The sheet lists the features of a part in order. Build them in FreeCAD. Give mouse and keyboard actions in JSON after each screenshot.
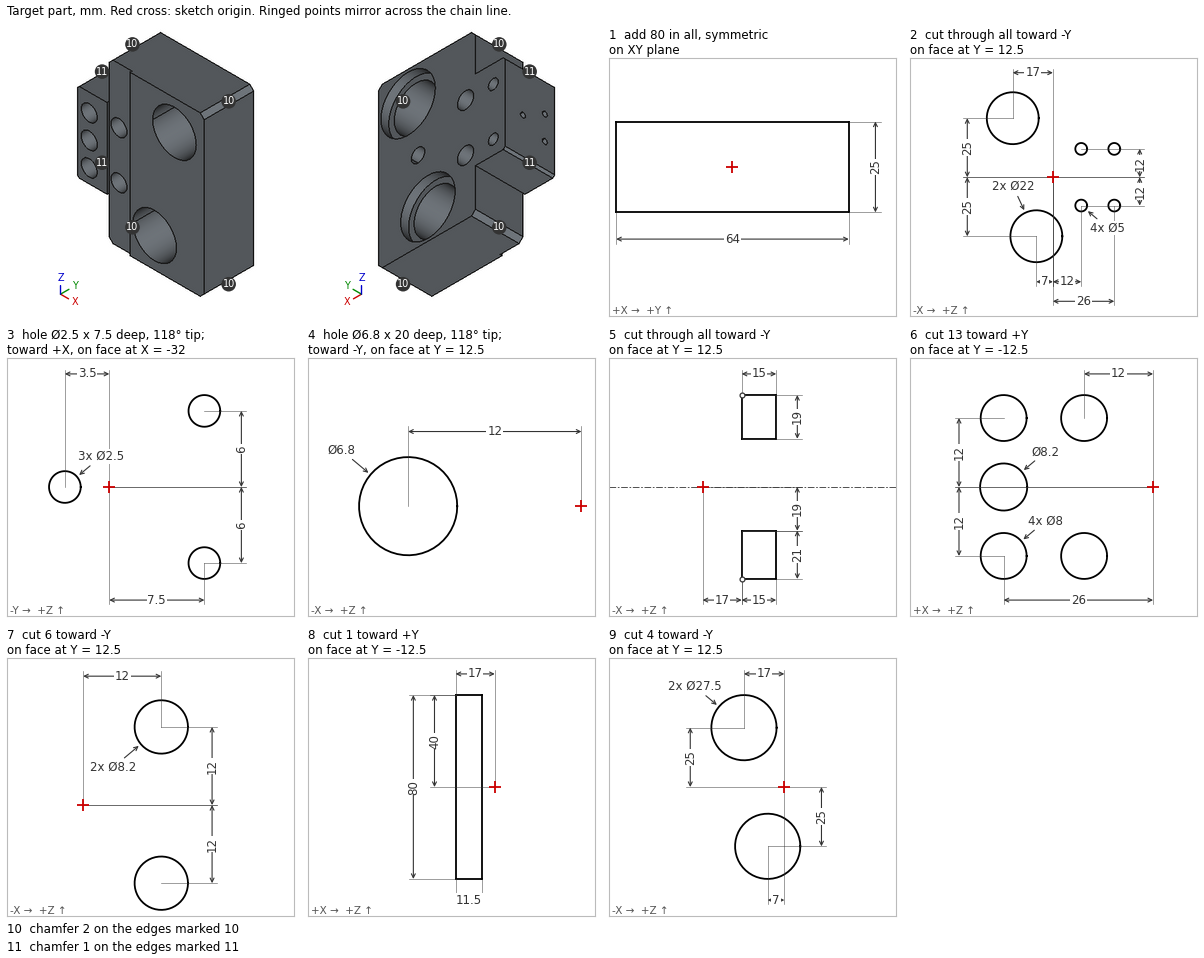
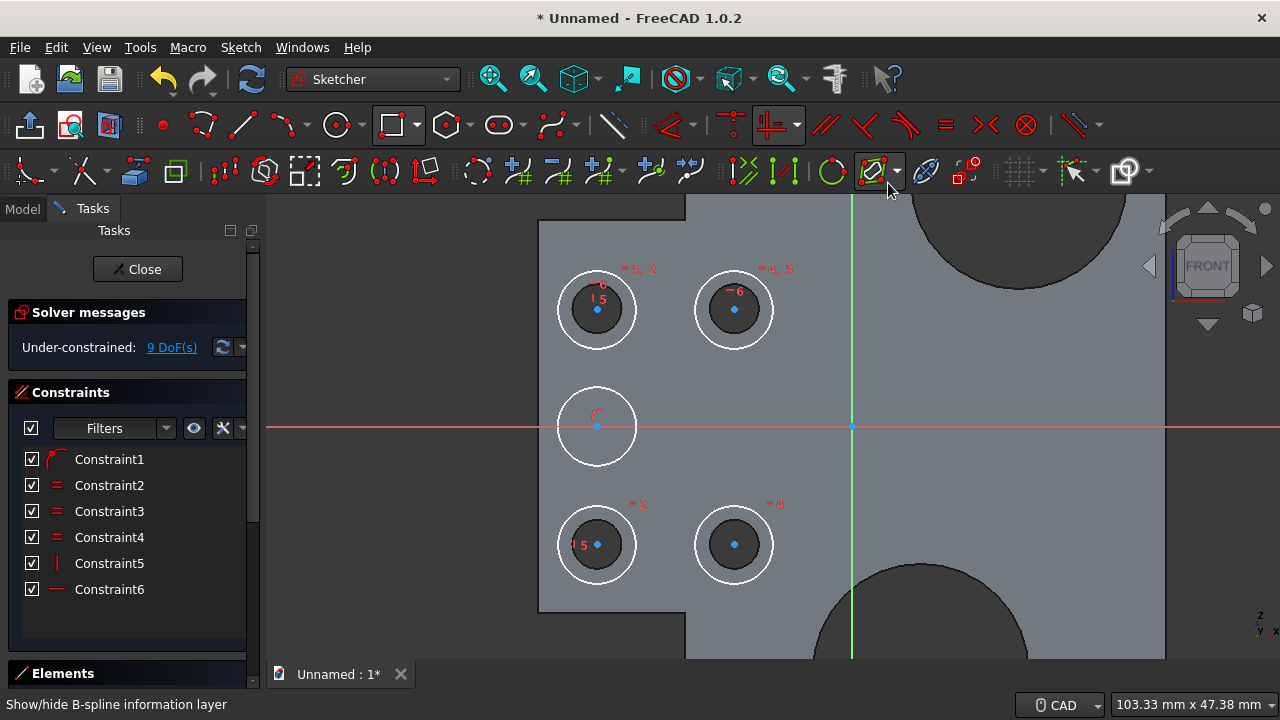
{"action": "left_click", "coordinate": [734, 310]}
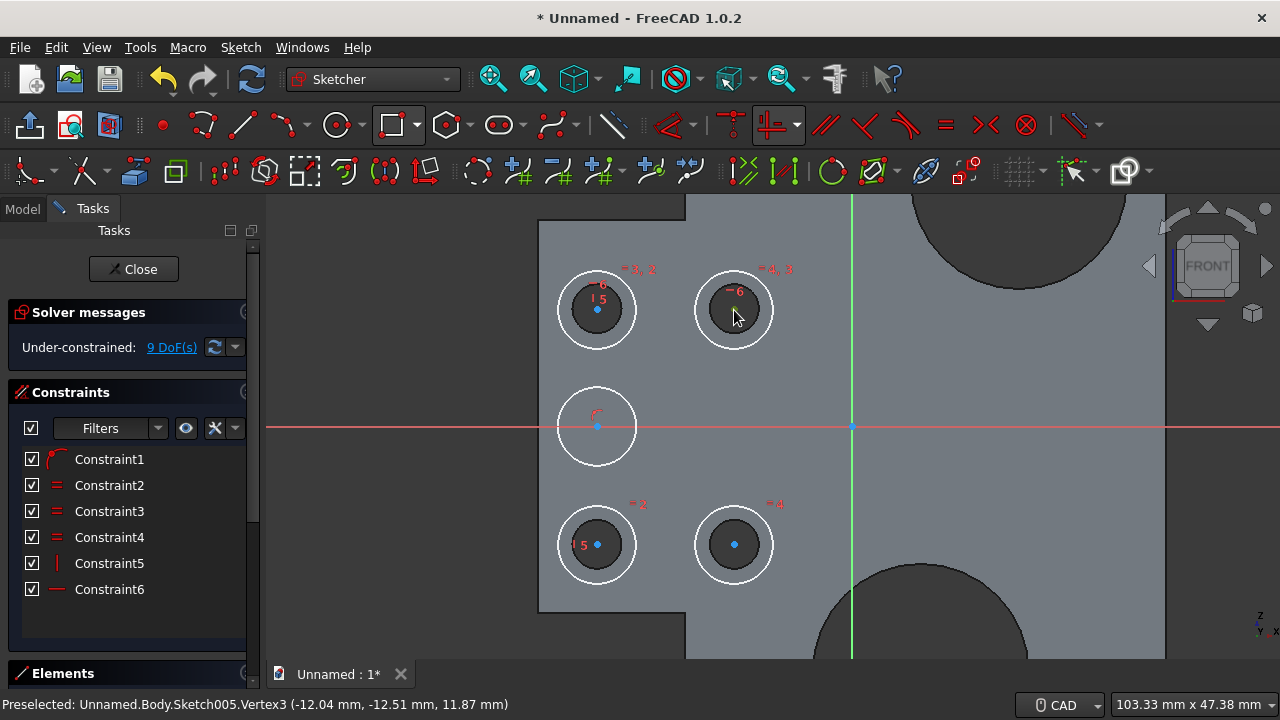
{"action": "left_click", "coordinate": [734, 545]}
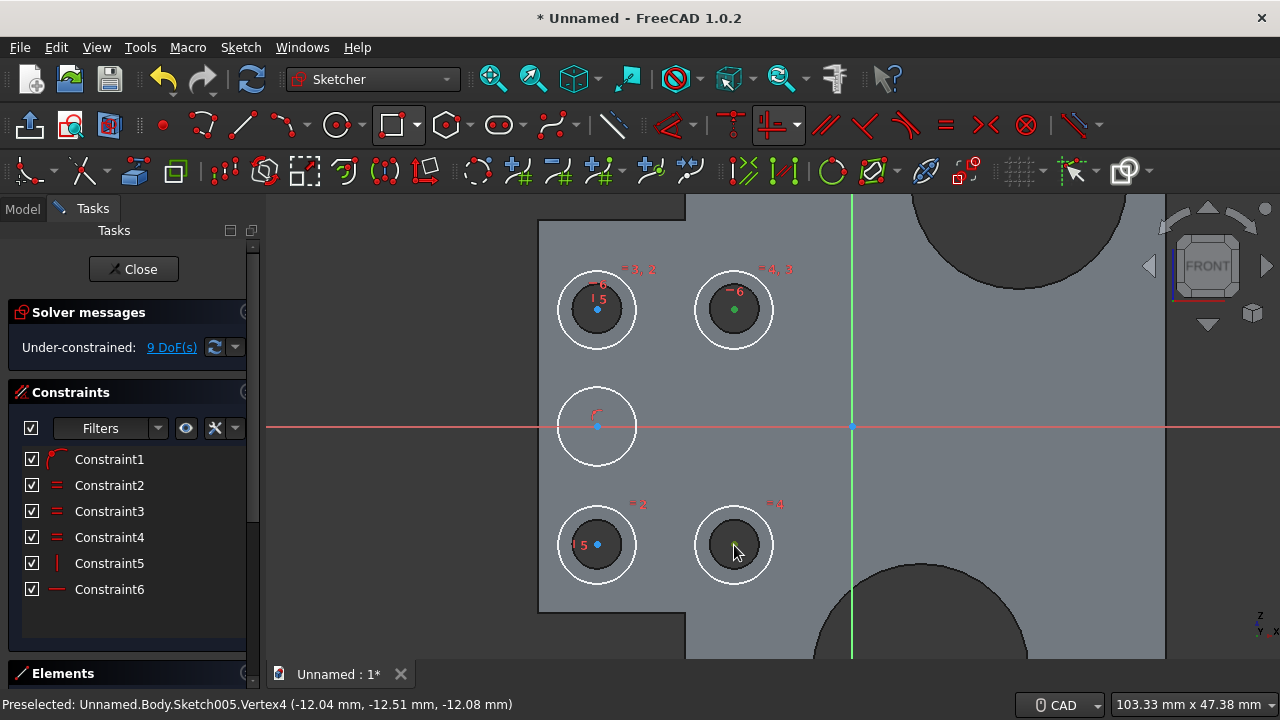
{"action": "left_click", "coordinate": [800, 126]}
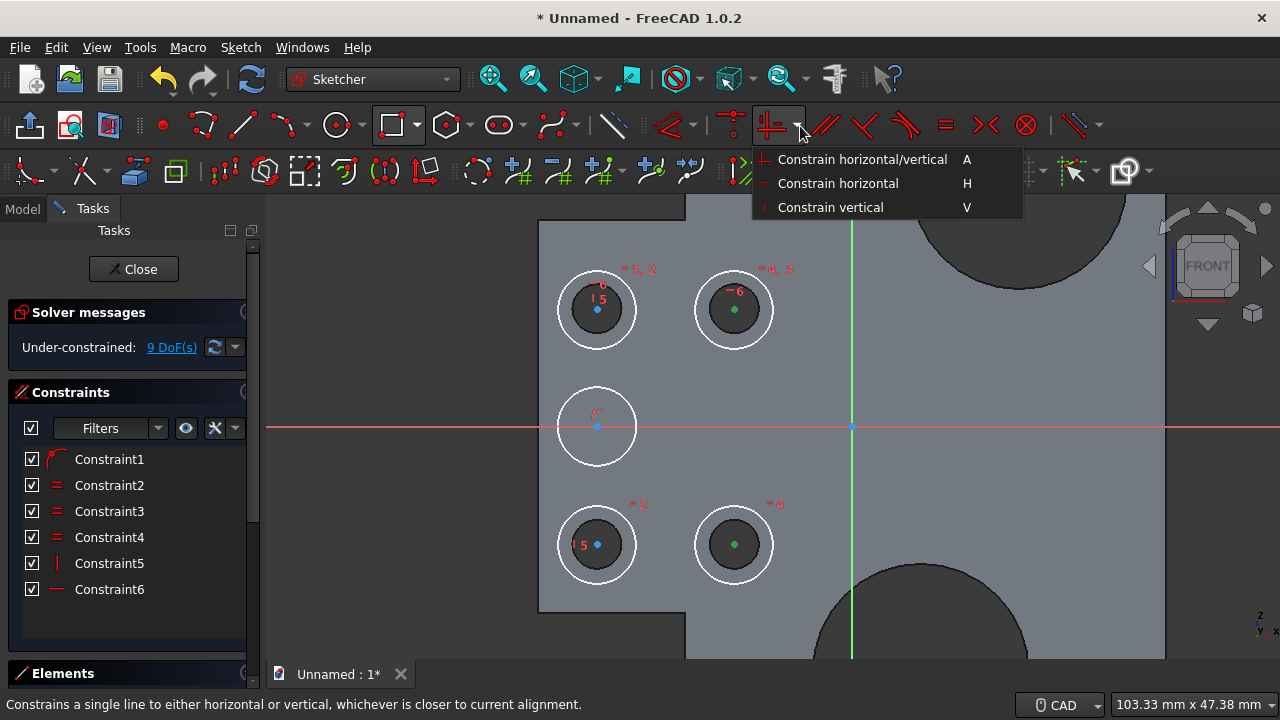
{"action": "left_click", "coordinate": [888, 207]}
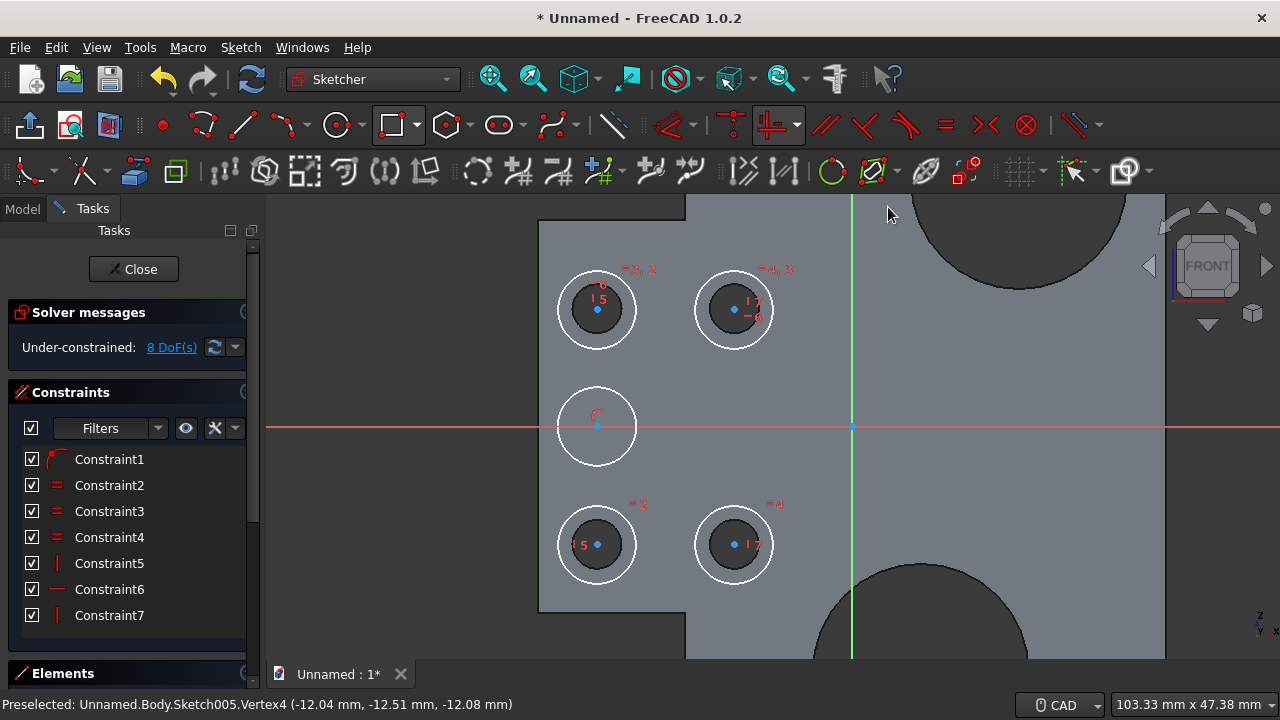
{"action": "left_click", "coordinate": [597, 545]}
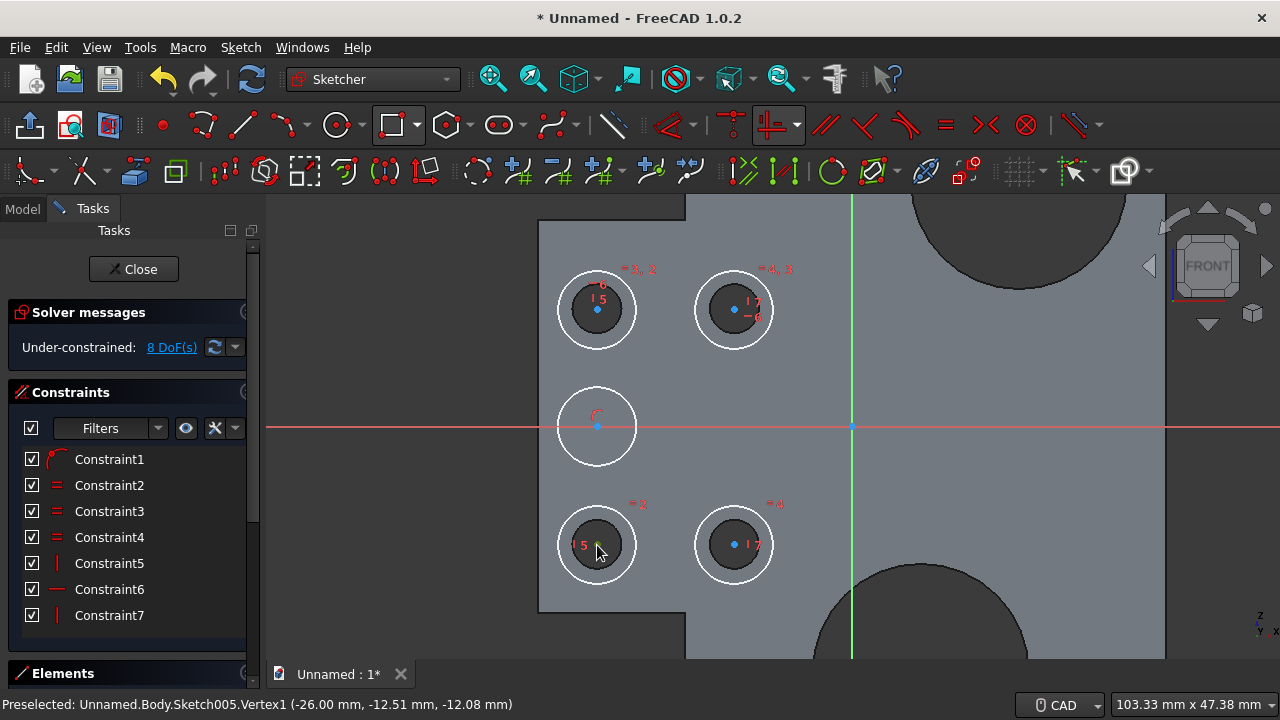
{"action": "left_click", "coordinate": [734, 545]}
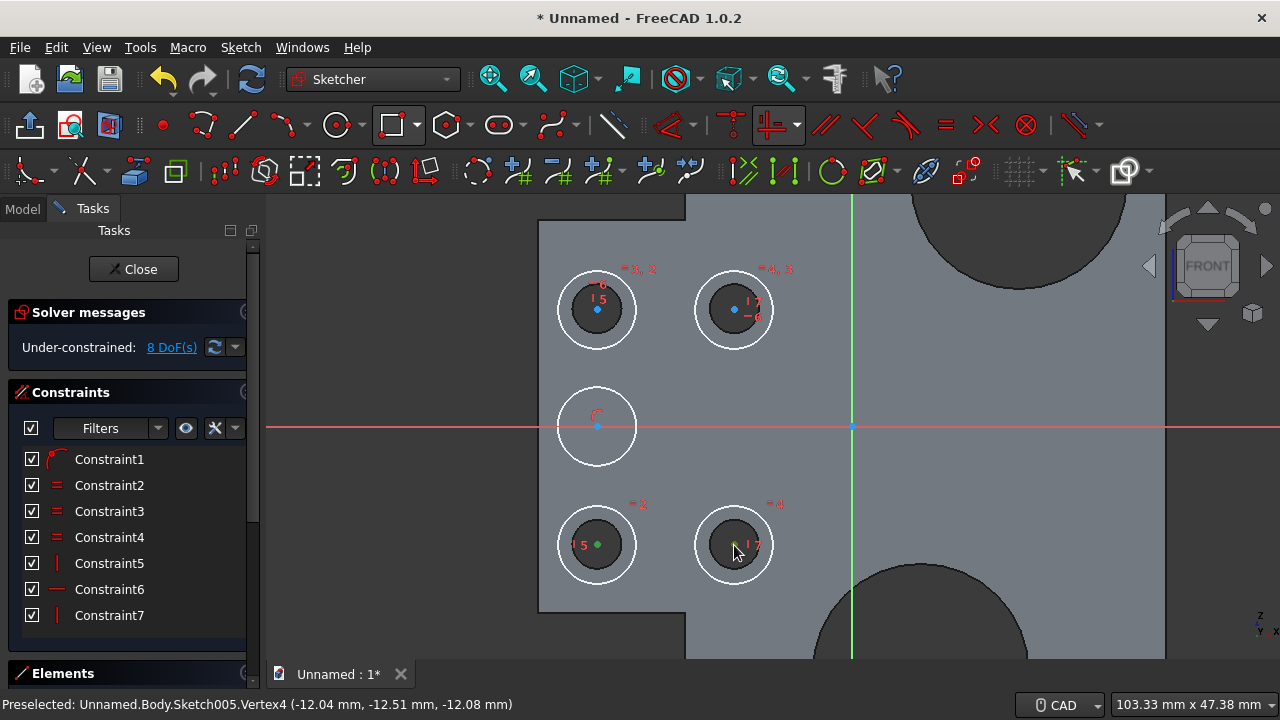
{"action": "left_click", "coordinate": [800, 126]}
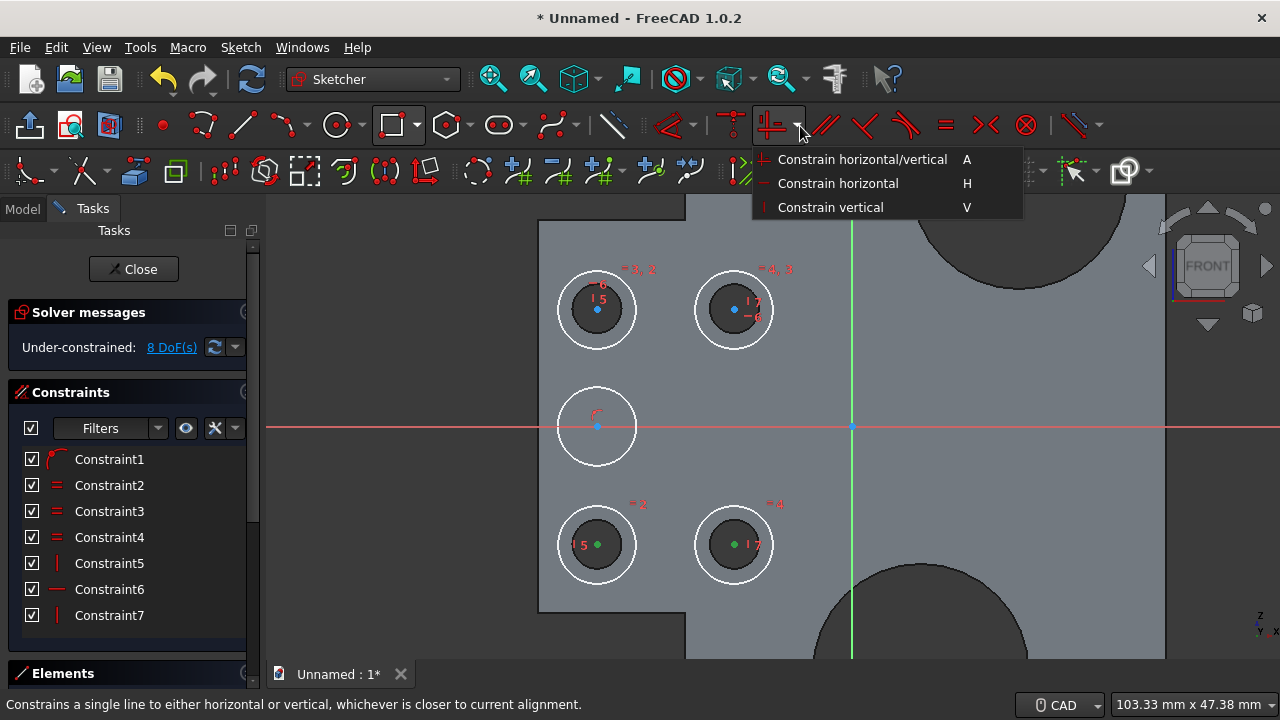
{"action": "left_click", "coordinate": [888, 183]}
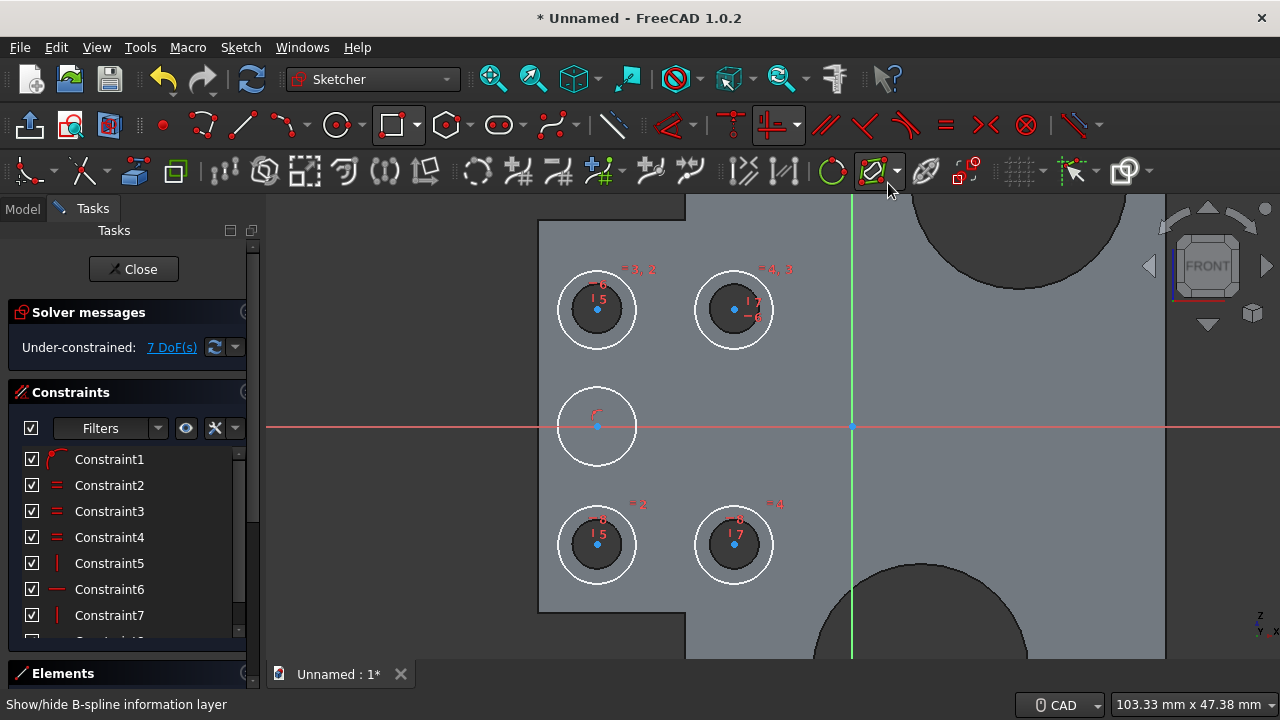
{"action": "left_click", "coordinate": [597, 545]}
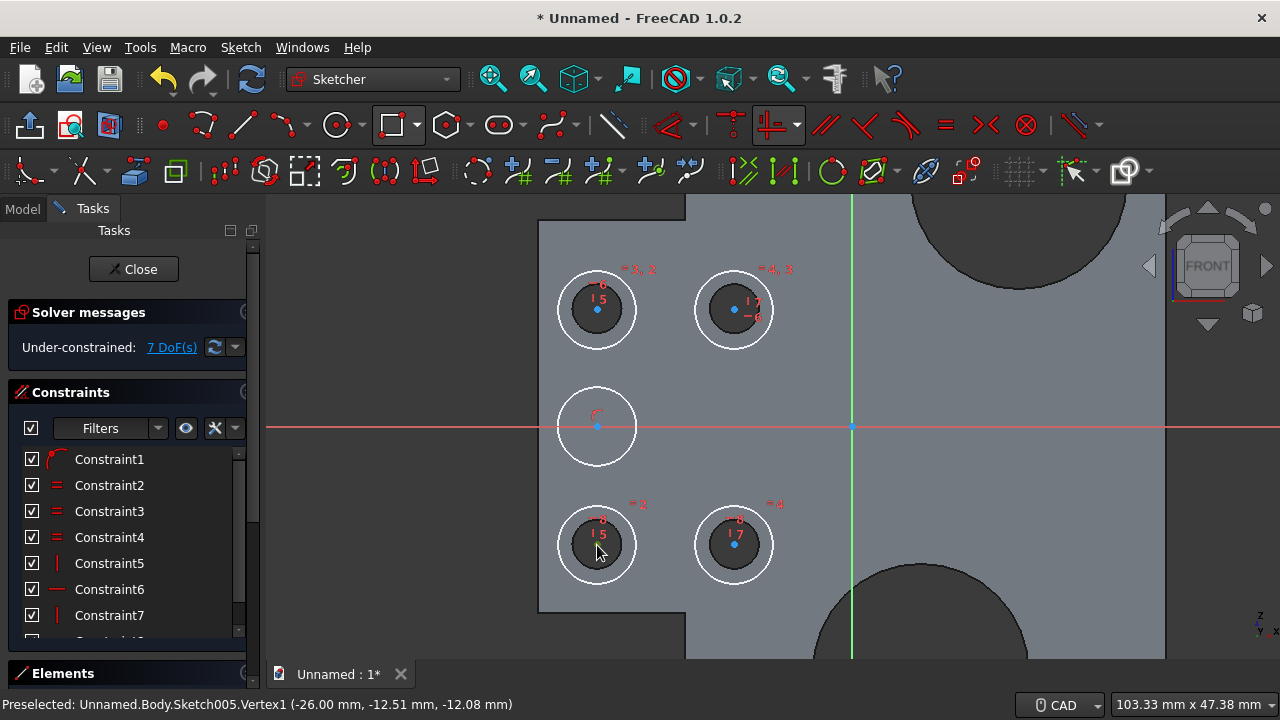
{"action": "left_click", "coordinate": [597, 426]}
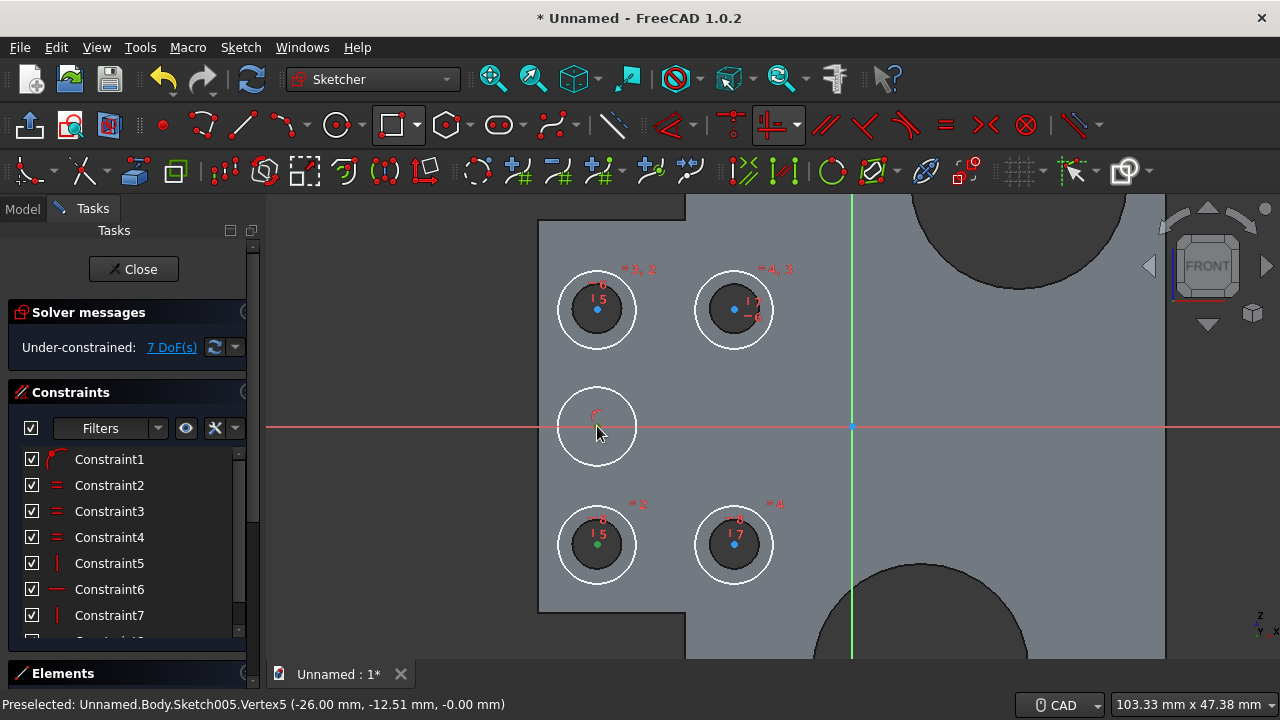
{"action": "left_click", "coordinate": [800, 126]}